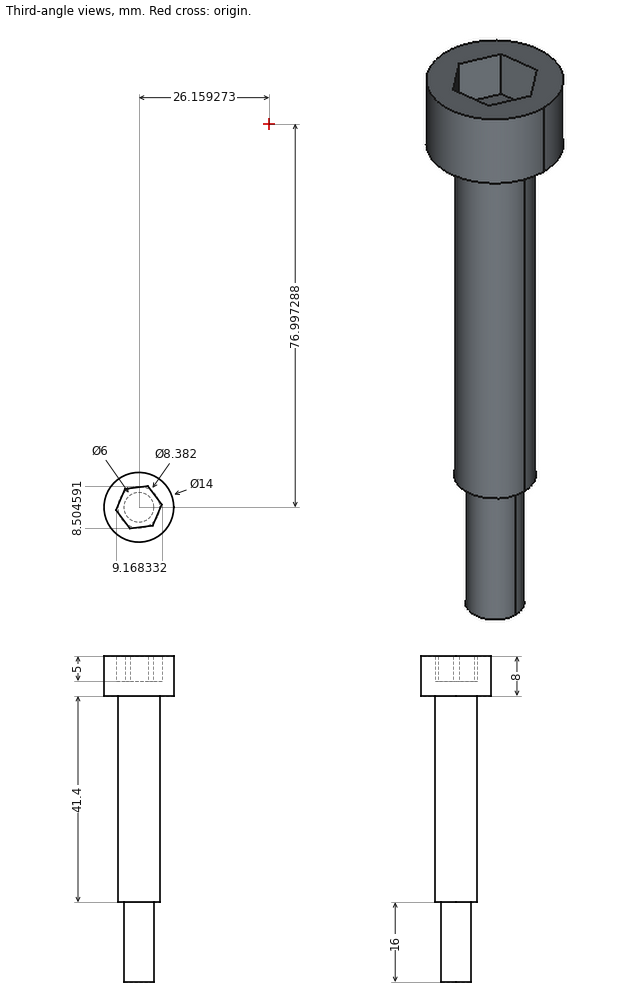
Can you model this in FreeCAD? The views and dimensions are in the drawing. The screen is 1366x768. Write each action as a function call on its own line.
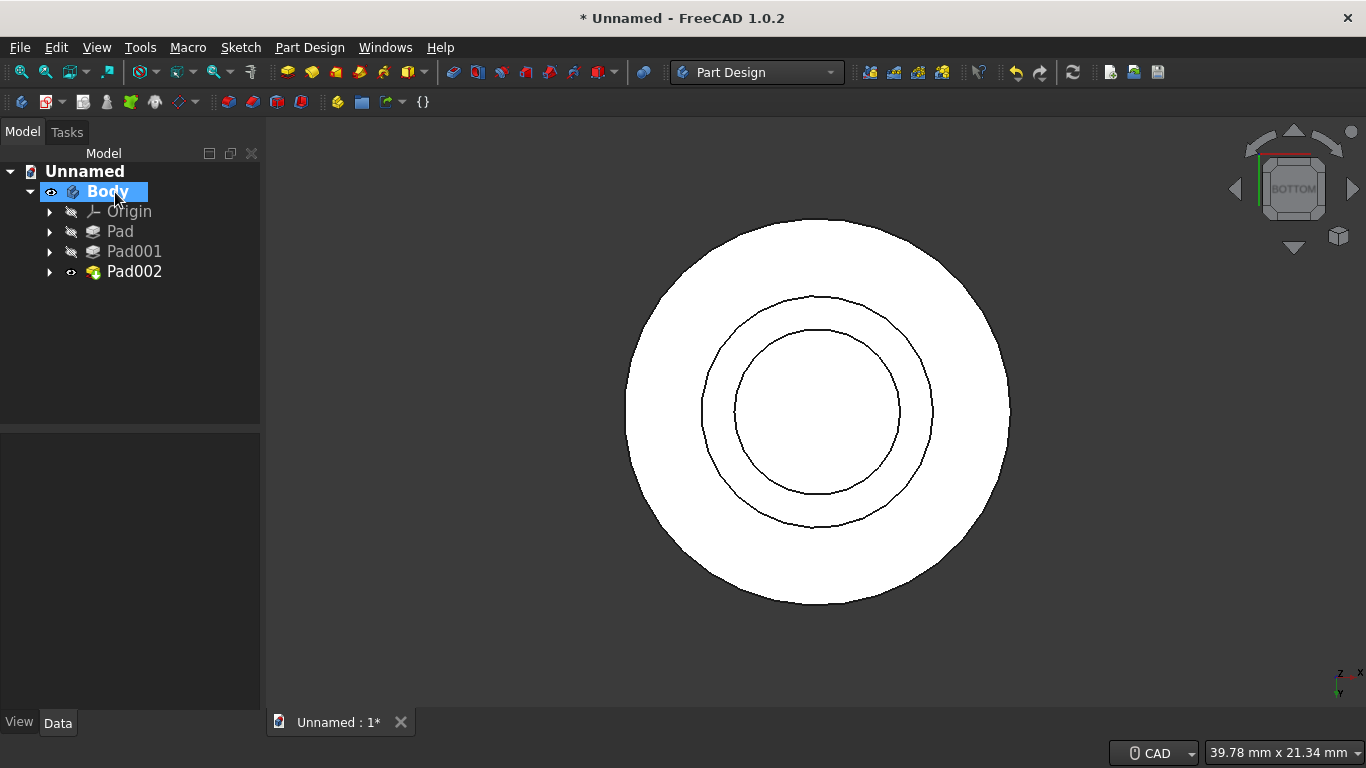
key(0)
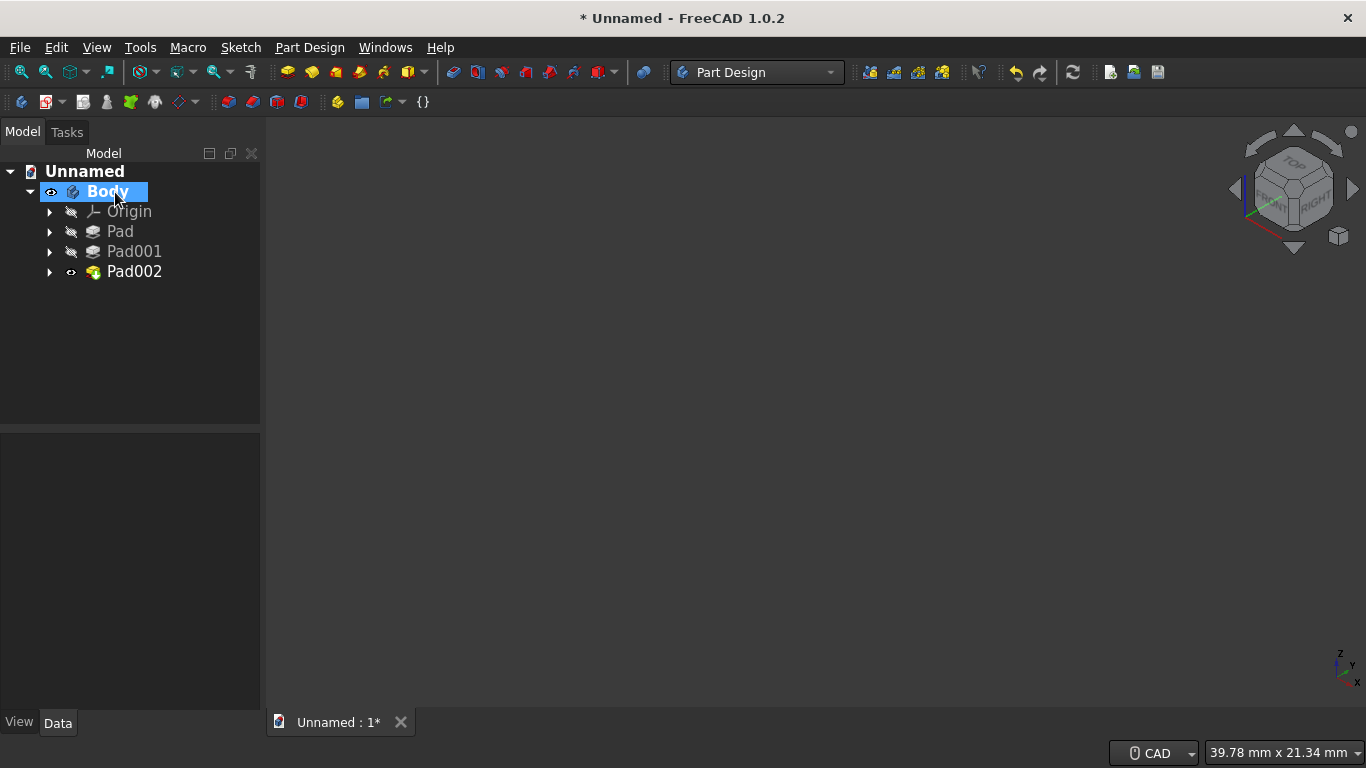
click(22, 72)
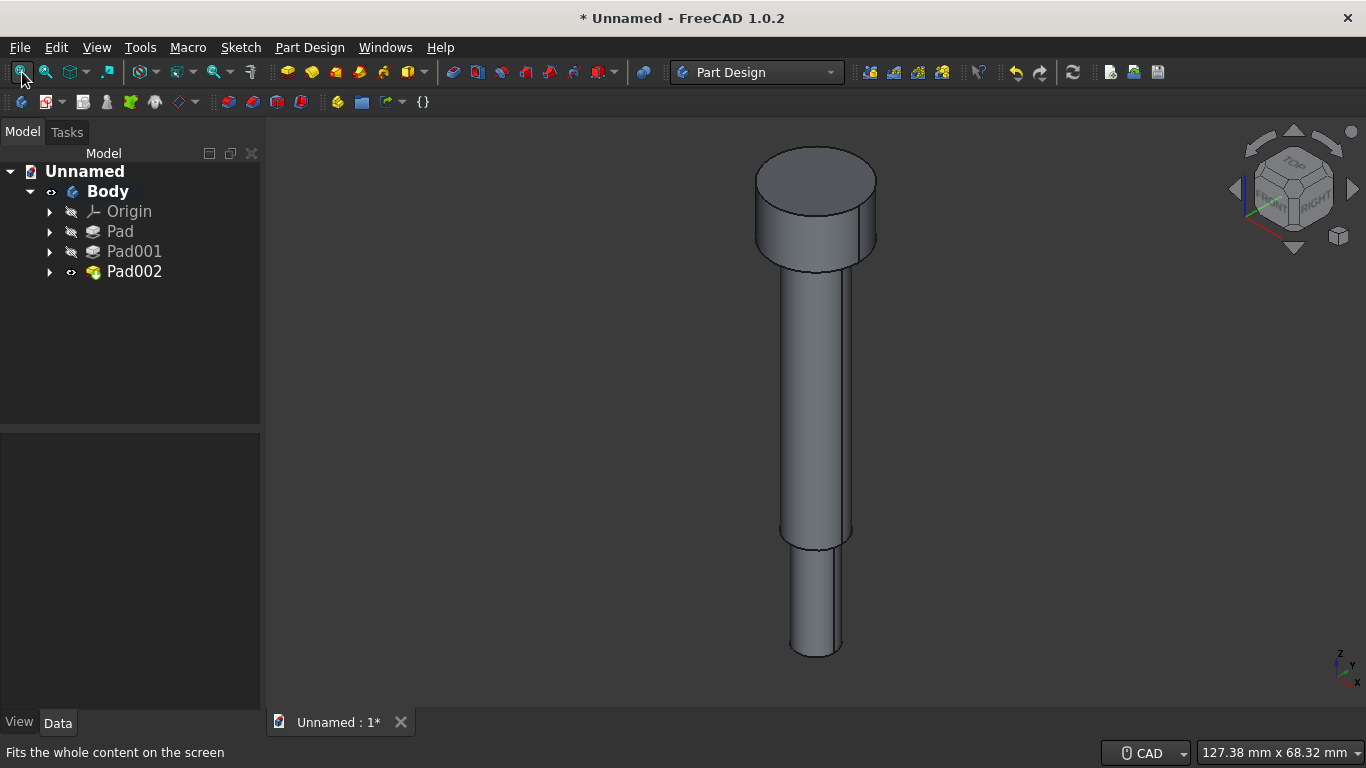
click(816, 180)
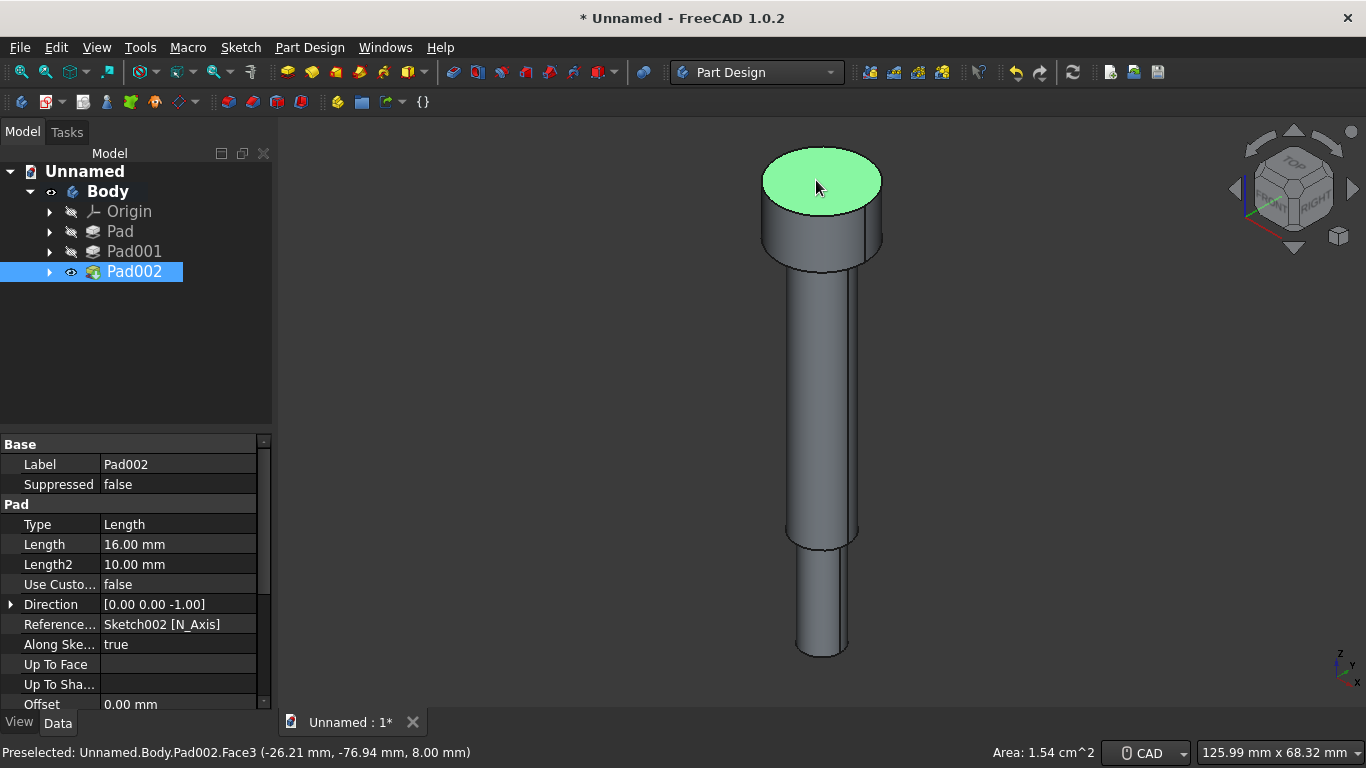
click(46, 102)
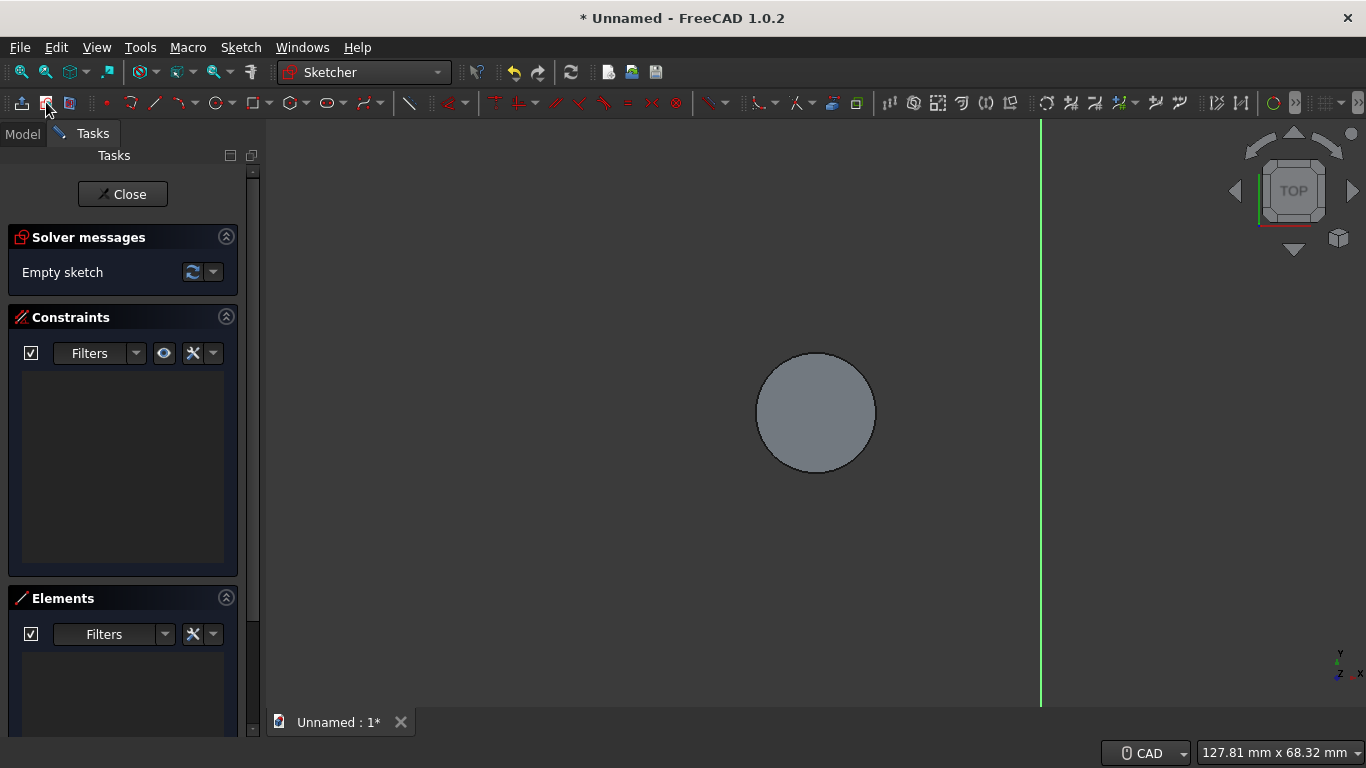
scroll(833, 413, up, 8)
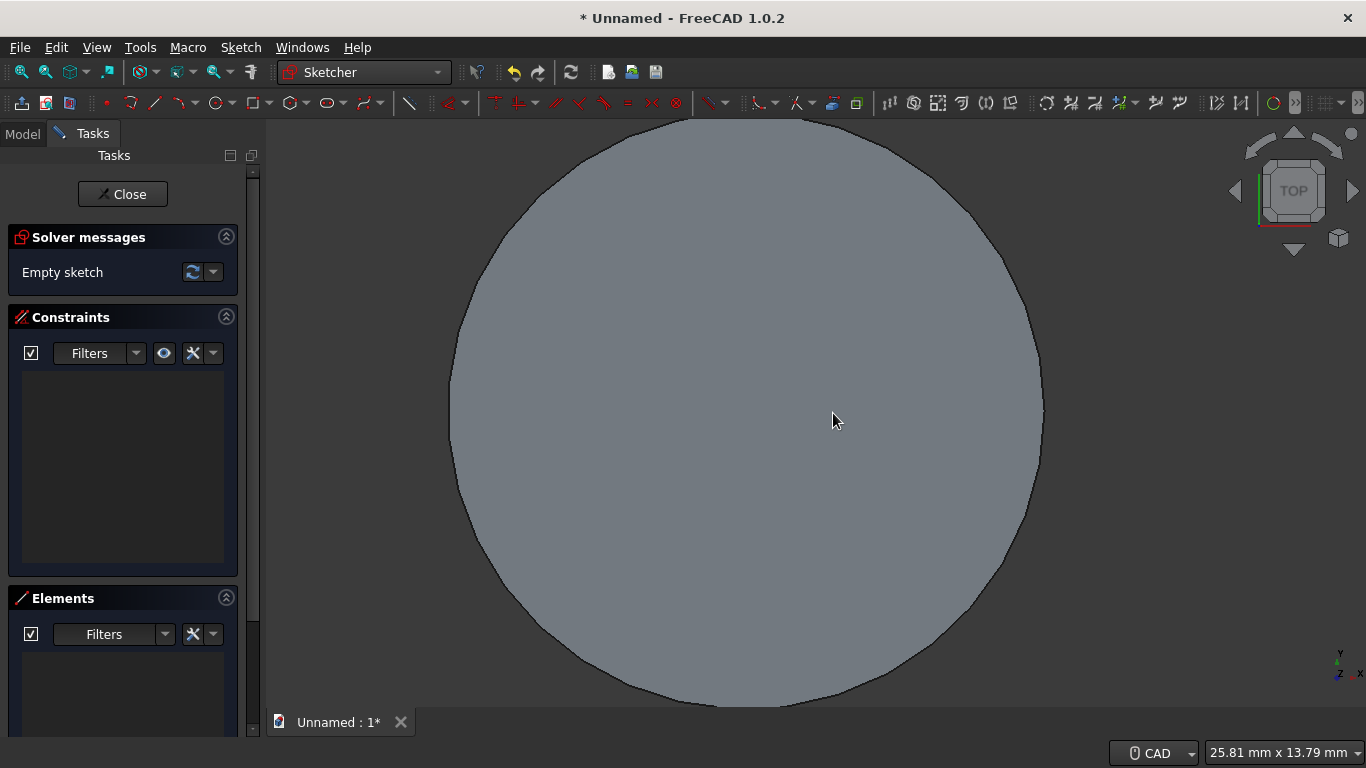
click(290, 104)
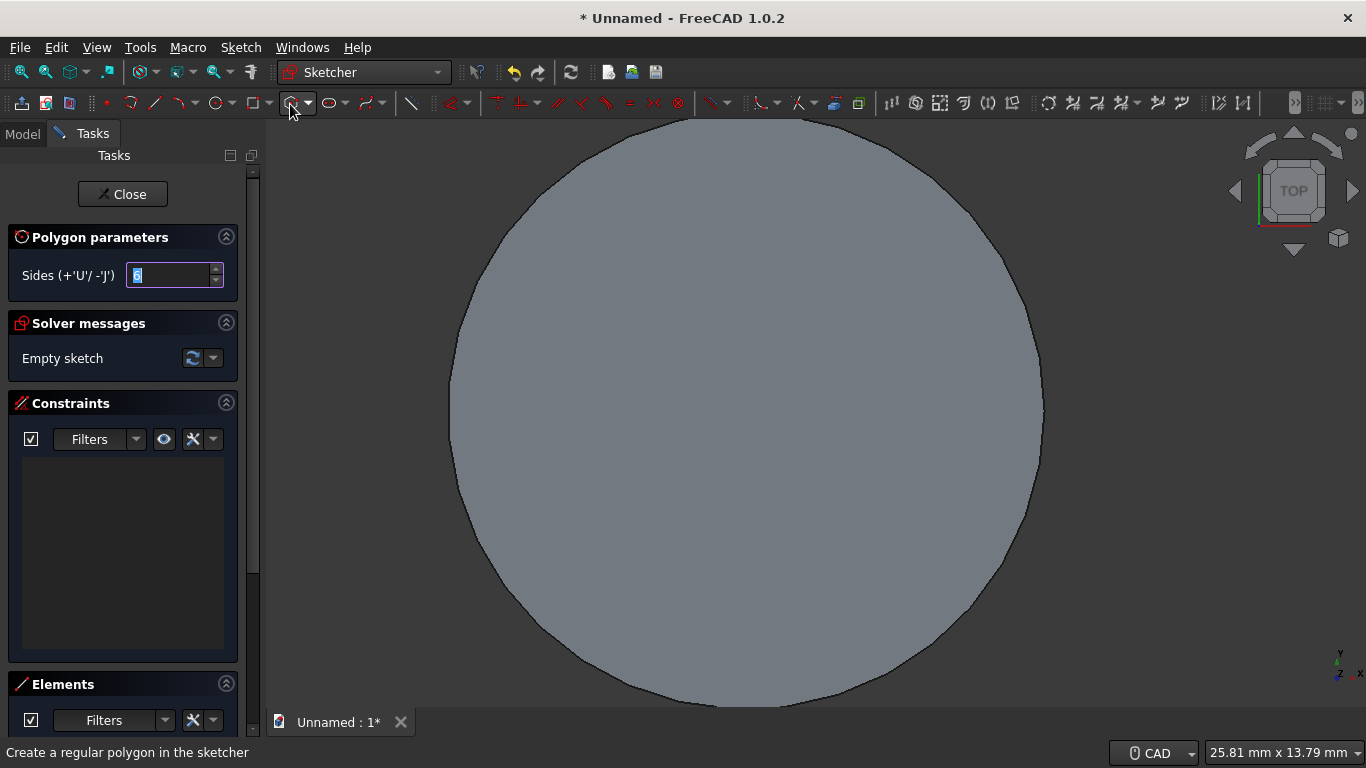
click(746, 411)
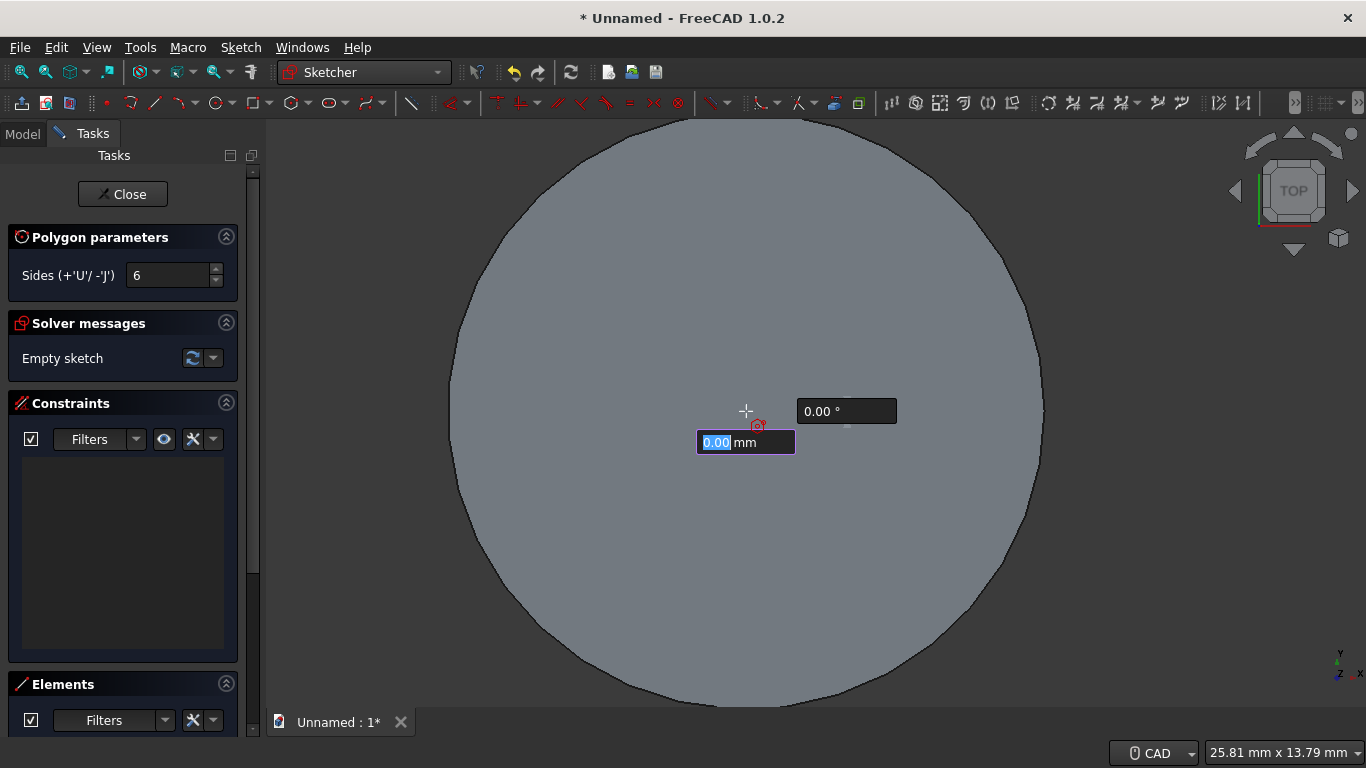
click(551, 435)
key(Escape)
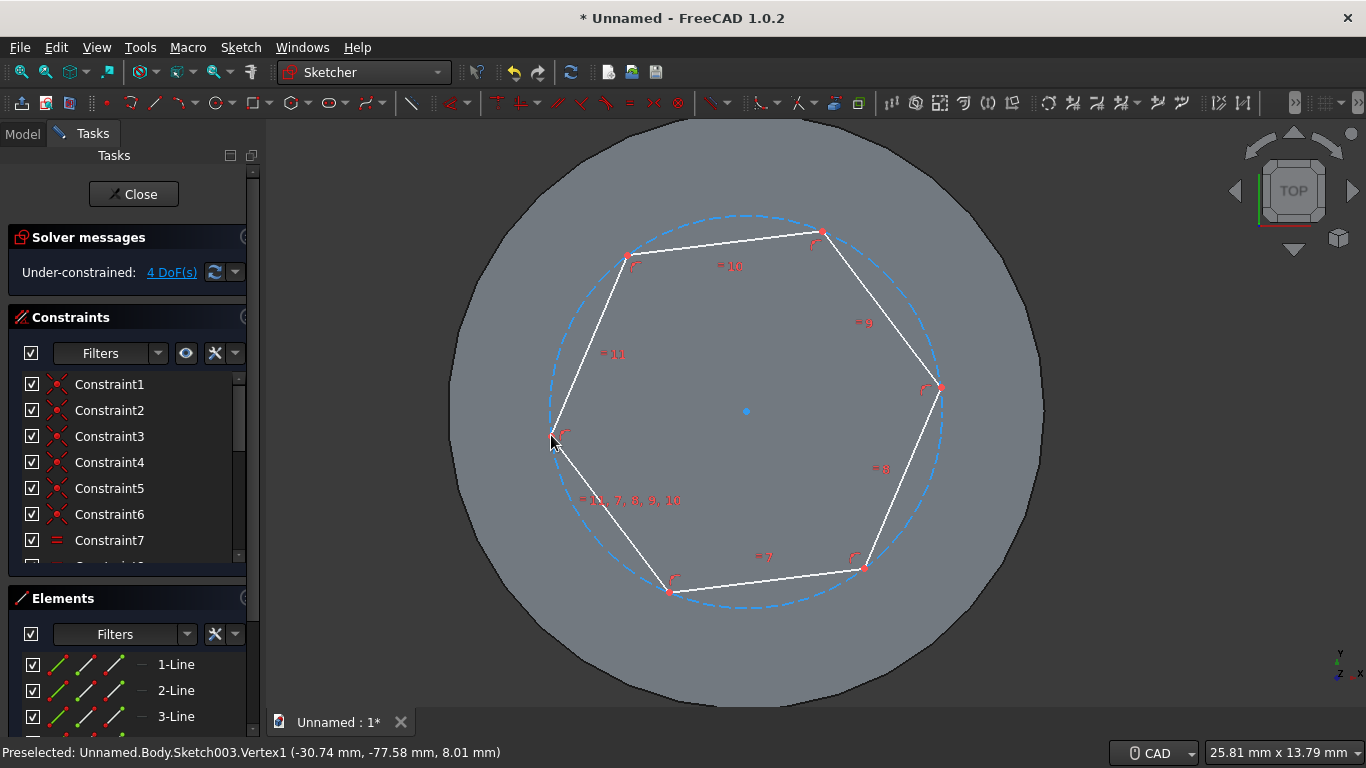
key(d)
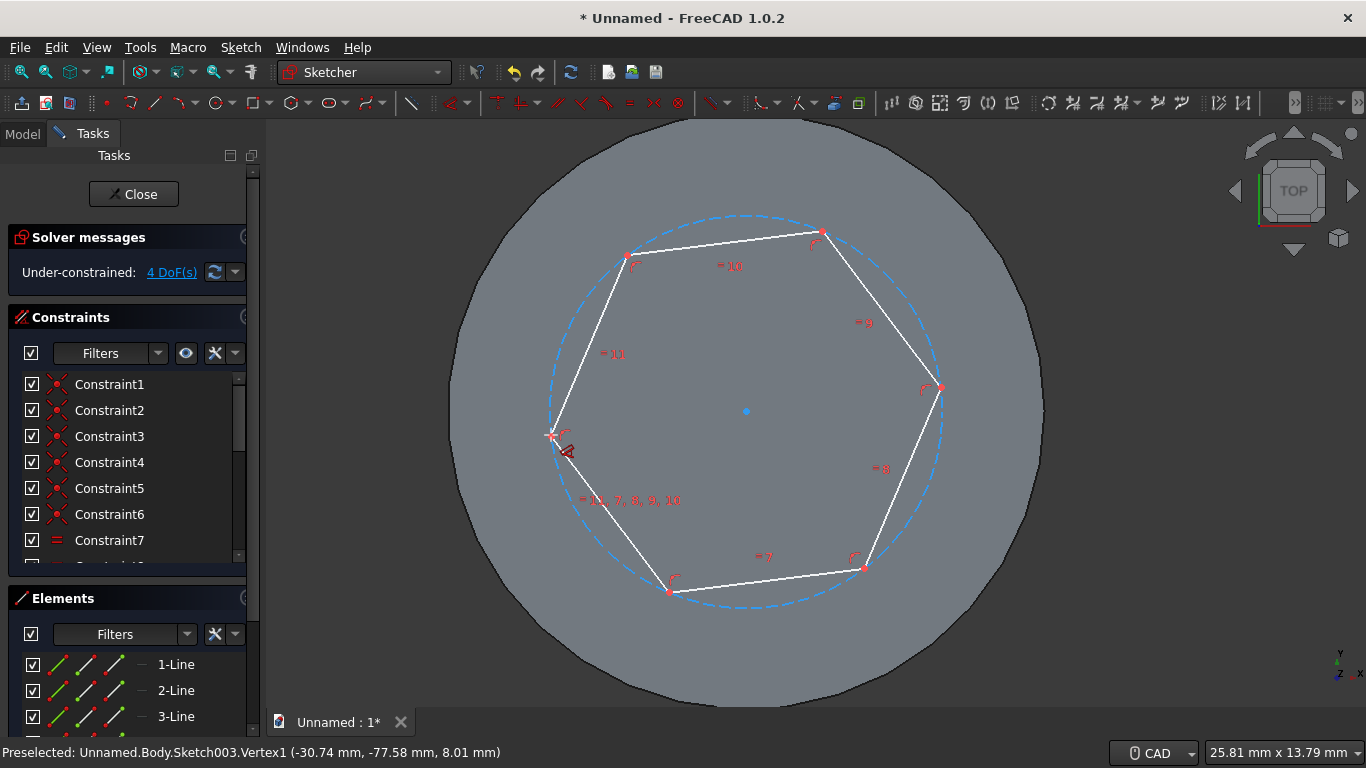
click(551, 436)